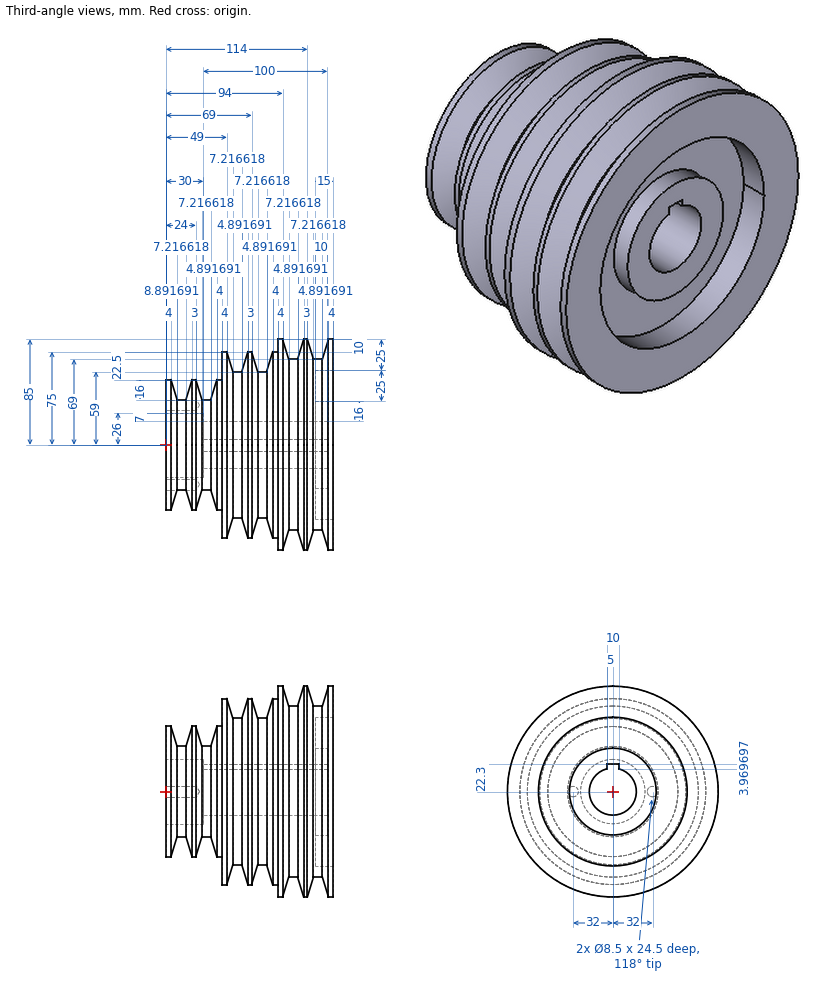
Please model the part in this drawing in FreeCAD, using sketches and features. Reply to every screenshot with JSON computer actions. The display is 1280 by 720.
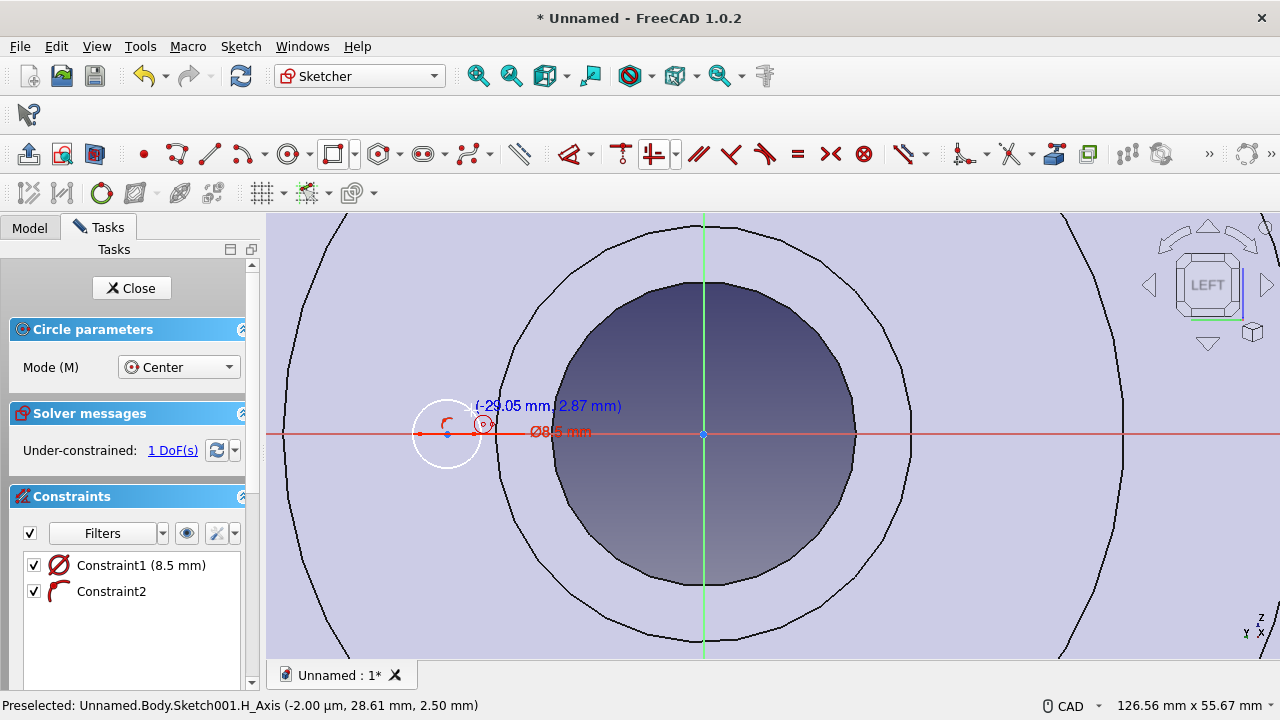
{"action": "left_click", "coordinate": [960, 434]}
{"action": "mouse_move", "coordinate": [984, 410]}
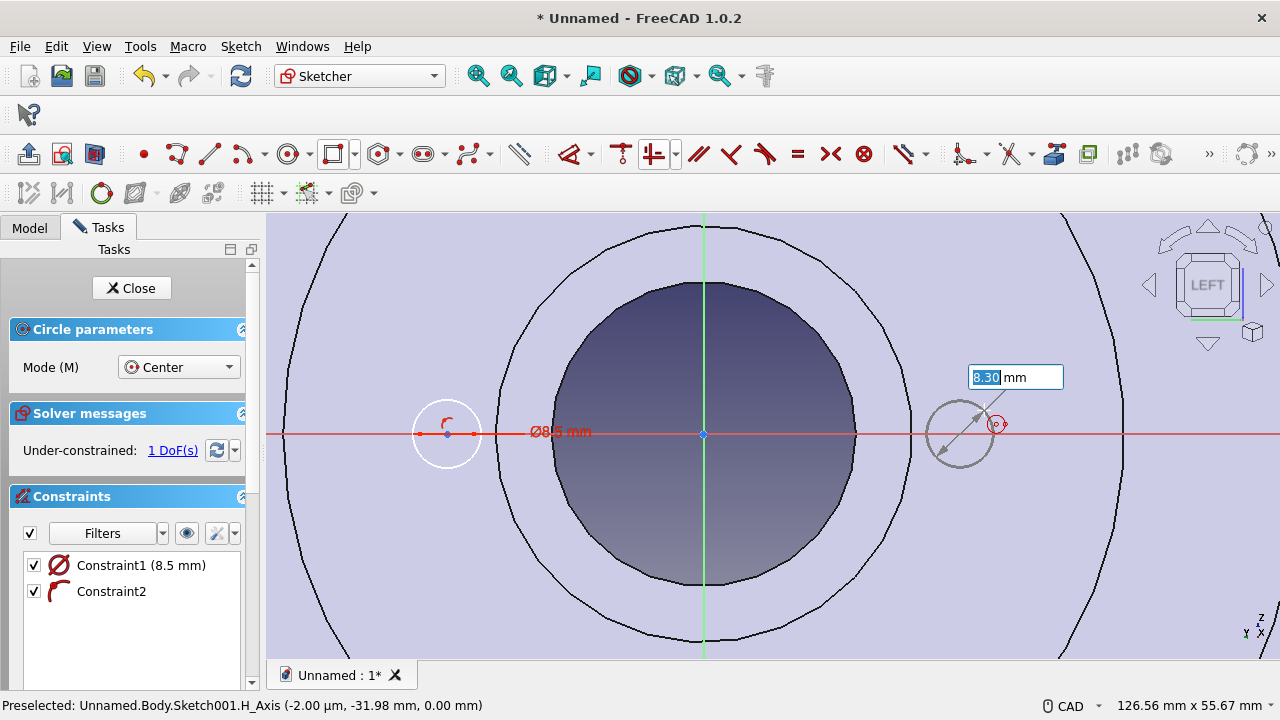
{"action": "type", "text": "8.5"}
{"action": "key", "text": "Return"}
{"action": "key", "text": "Escape"}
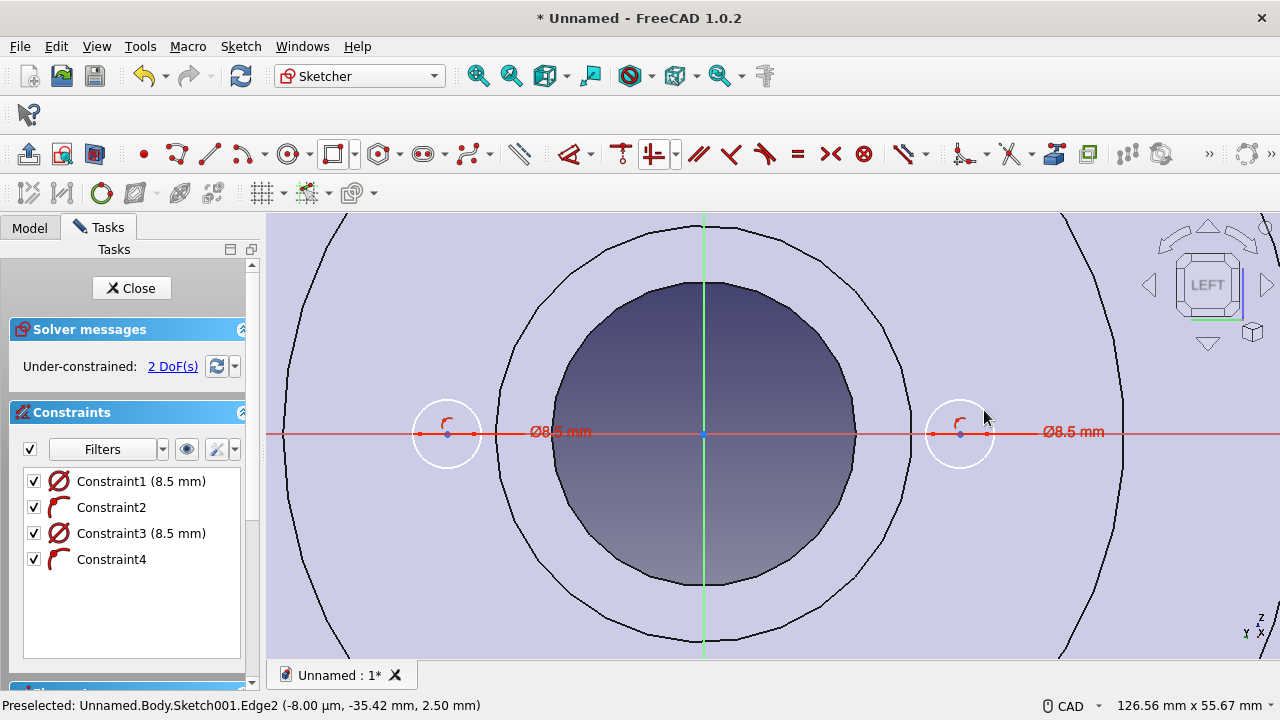
{"action": "left_click", "coordinate": [568, 154]}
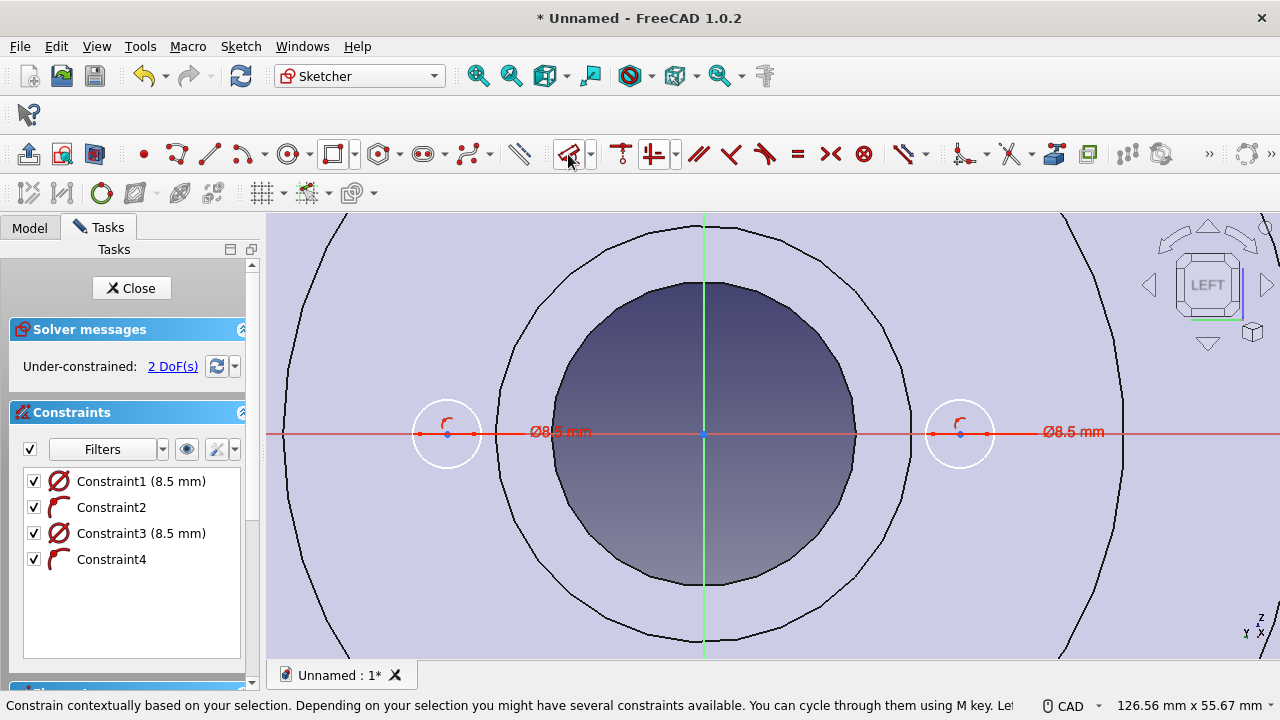
{"action": "left_click", "coordinate": [447, 434]}
{"action": "left_click", "coordinate": [575, 468]}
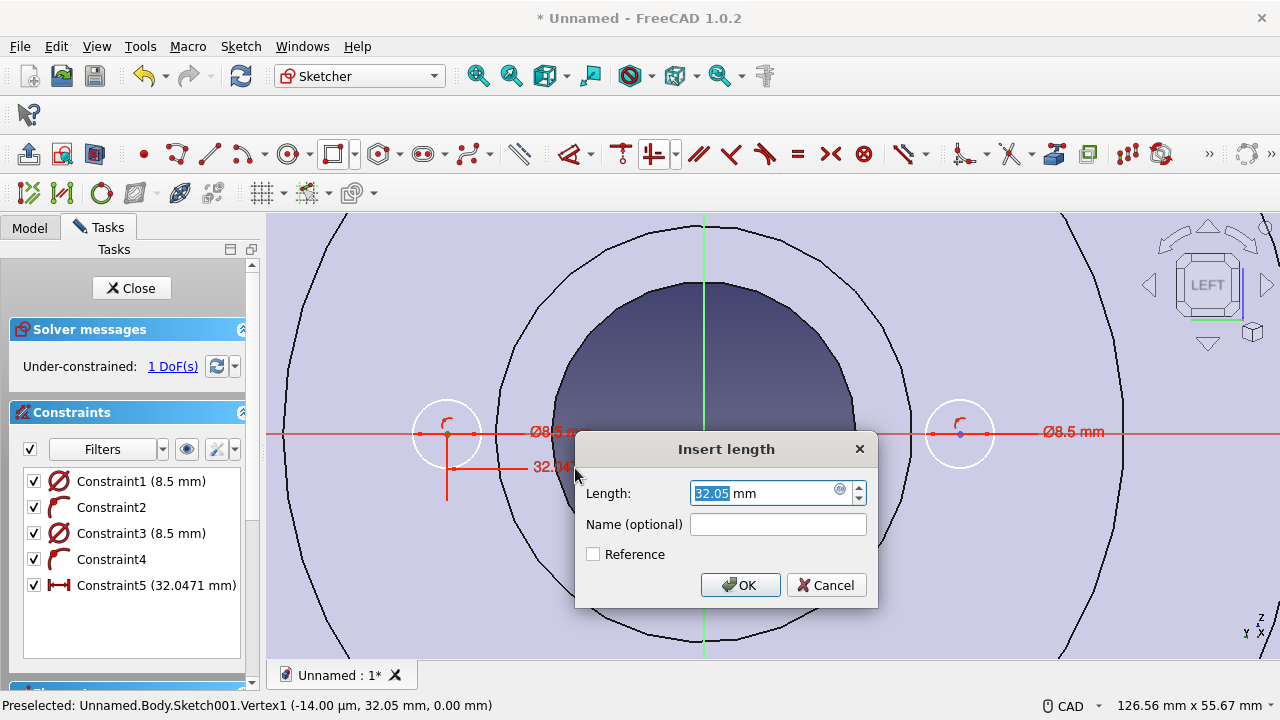
{"action": "type", "text": "32"}
{"action": "key", "text": "Return"}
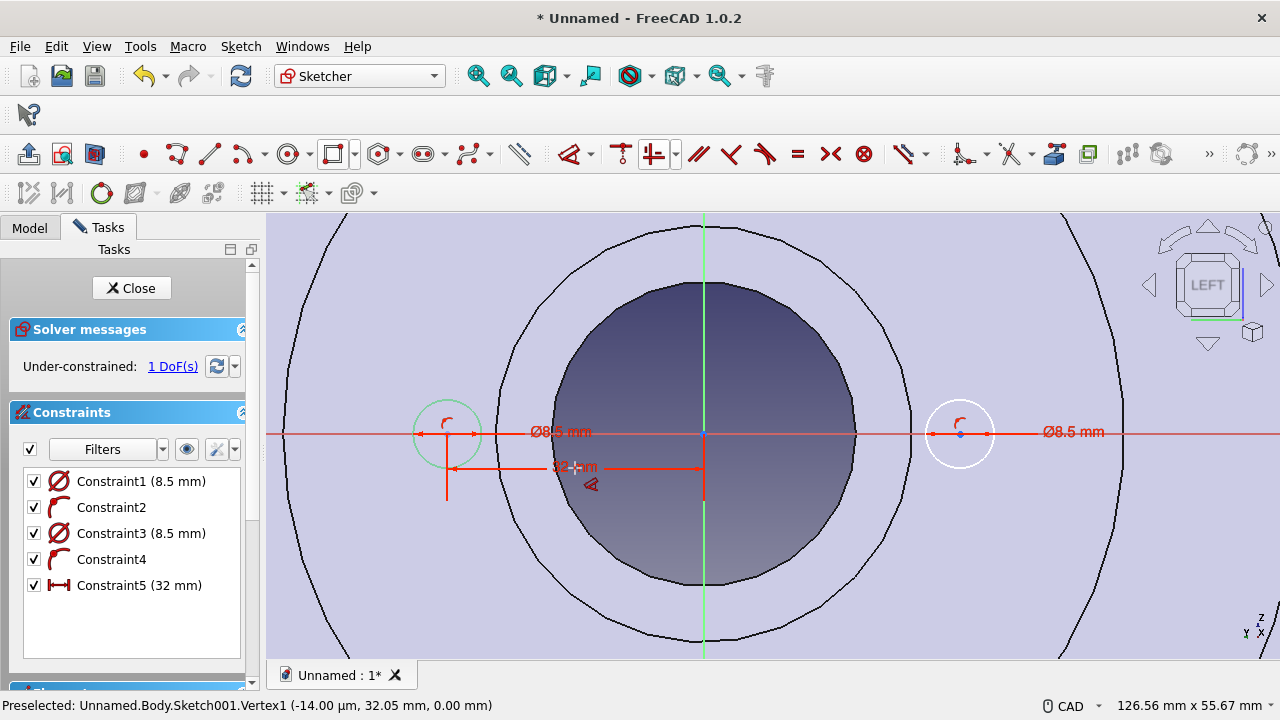
{"action": "left_click", "coordinate": [960, 434]}
{"action": "left_click", "coordinate": [832, 468]}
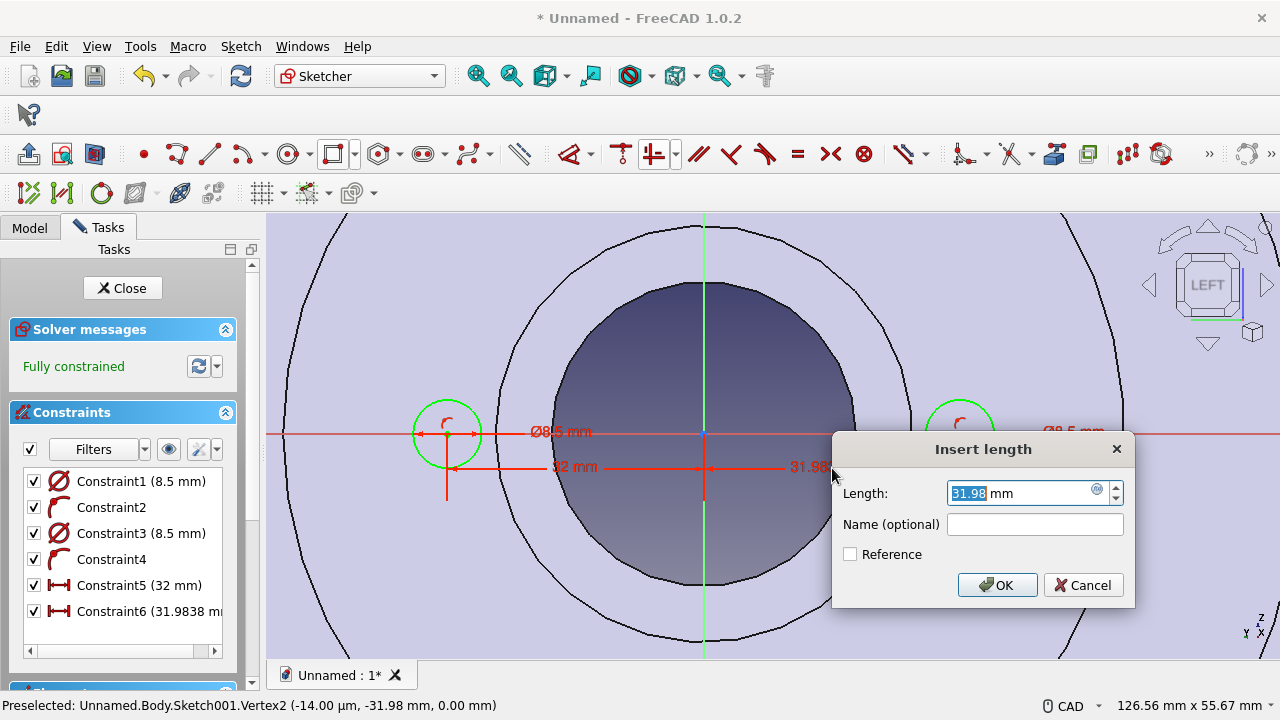
{"action": "type", "text": "32"}
{"action": "key", "text": "Return"}
{"action": "key", "text": "Escape"}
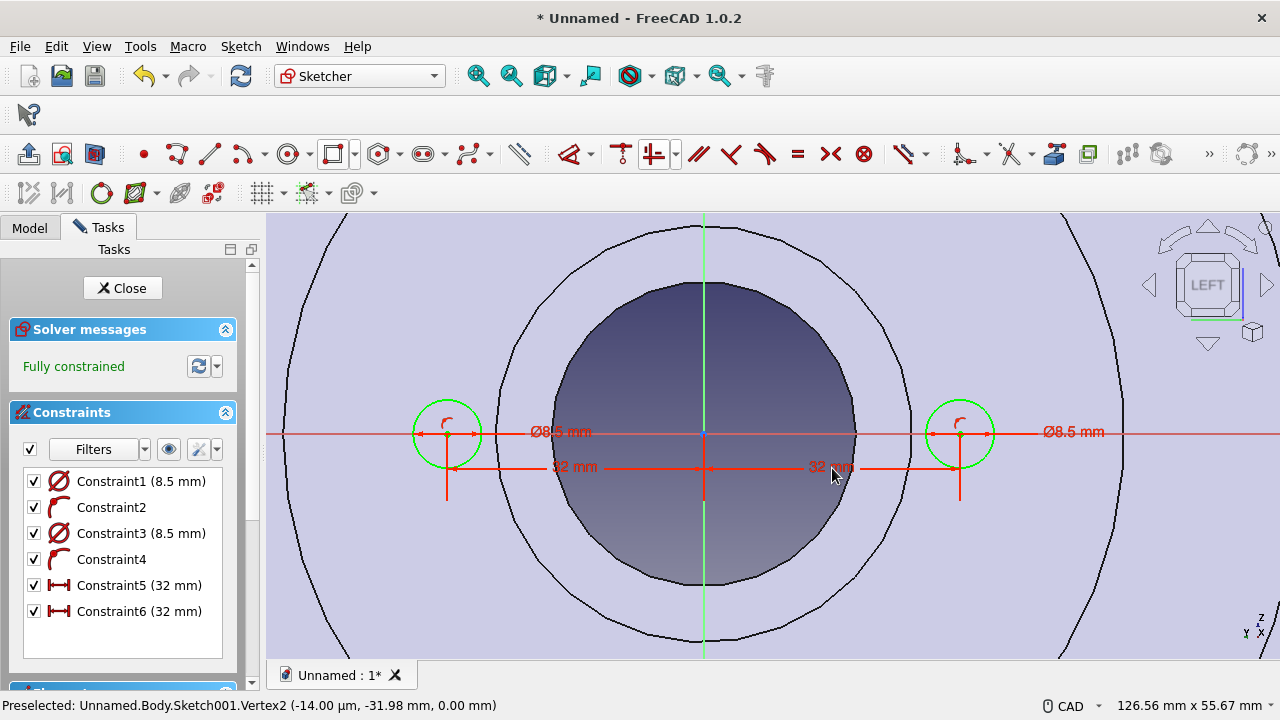
{"action": "left_click", "coordinate": [123, 288]}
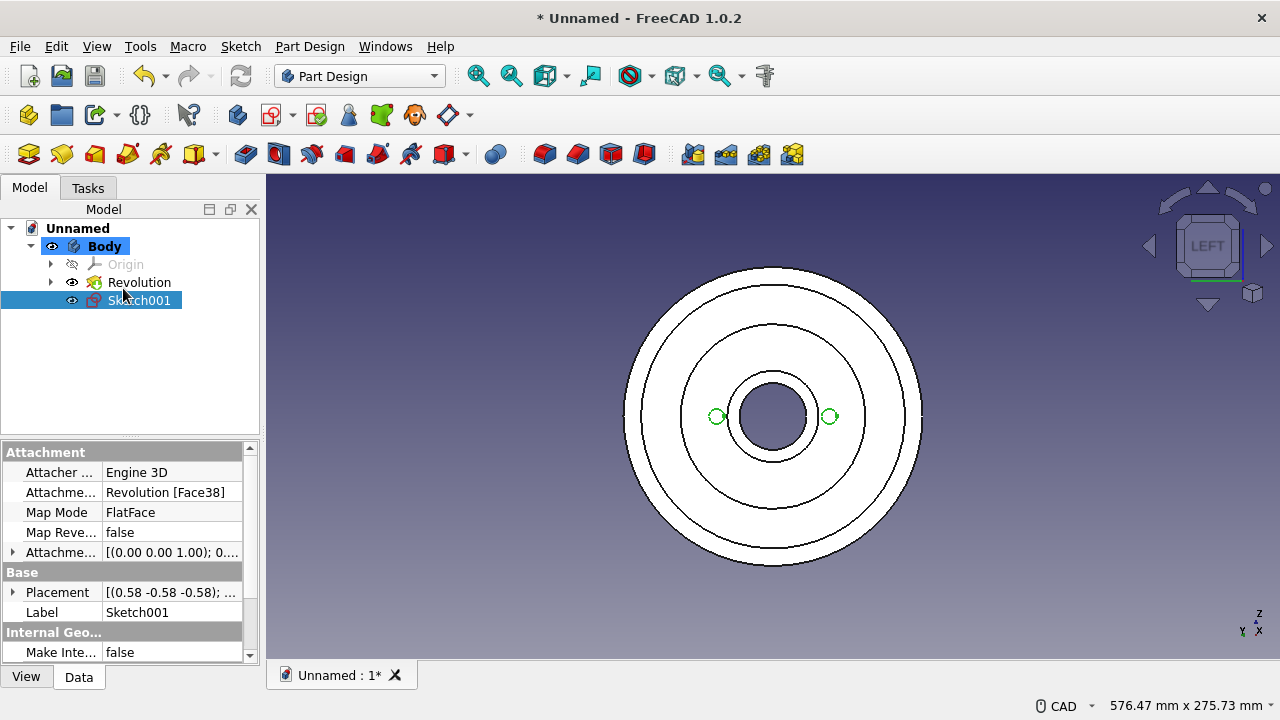
{"action": "left_click", "coordinate": [279, 154]}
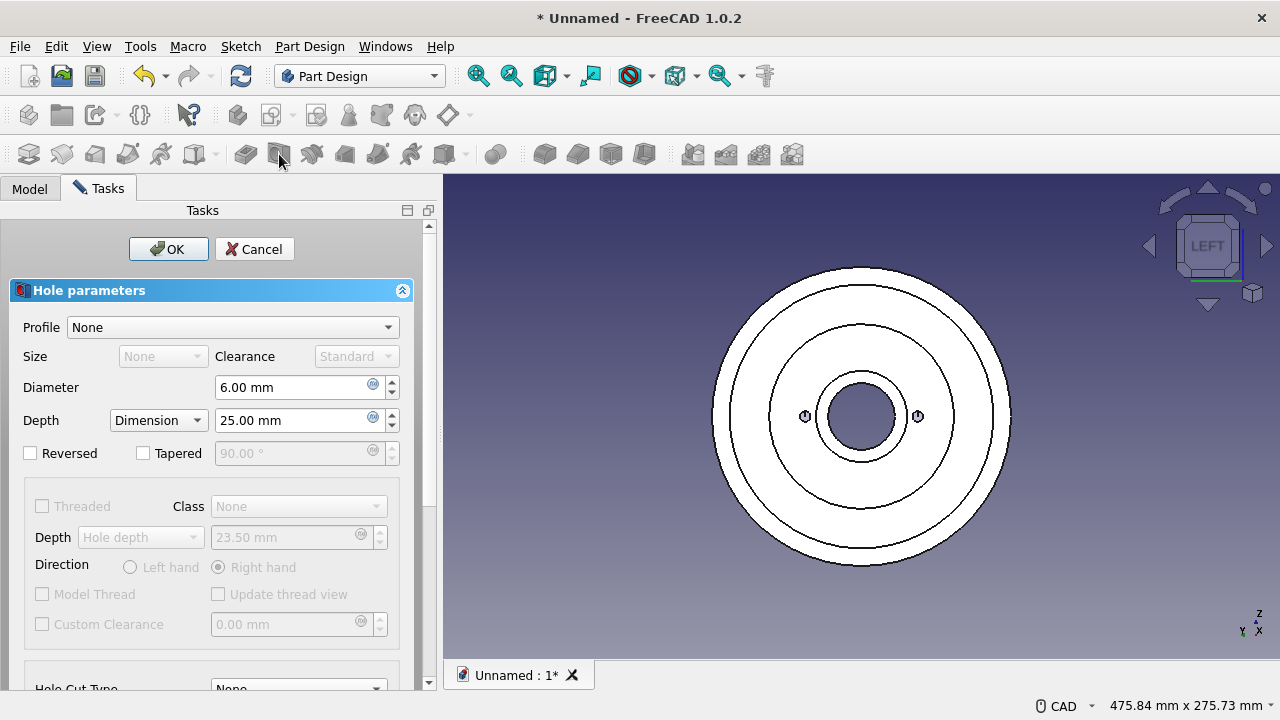
{"action": "triple_click", "coordinate": [300, 388]}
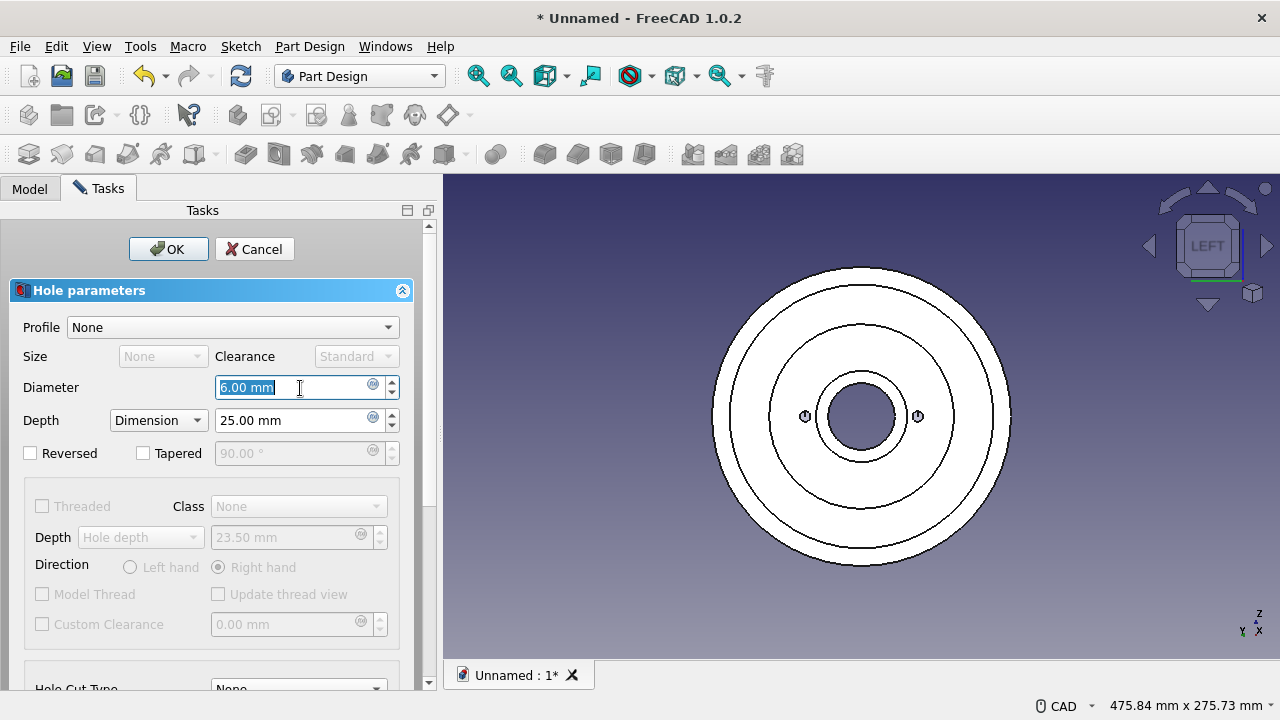
{"action": "type", "text": "8.5"}
{"action": "key", "text": "Tab"}